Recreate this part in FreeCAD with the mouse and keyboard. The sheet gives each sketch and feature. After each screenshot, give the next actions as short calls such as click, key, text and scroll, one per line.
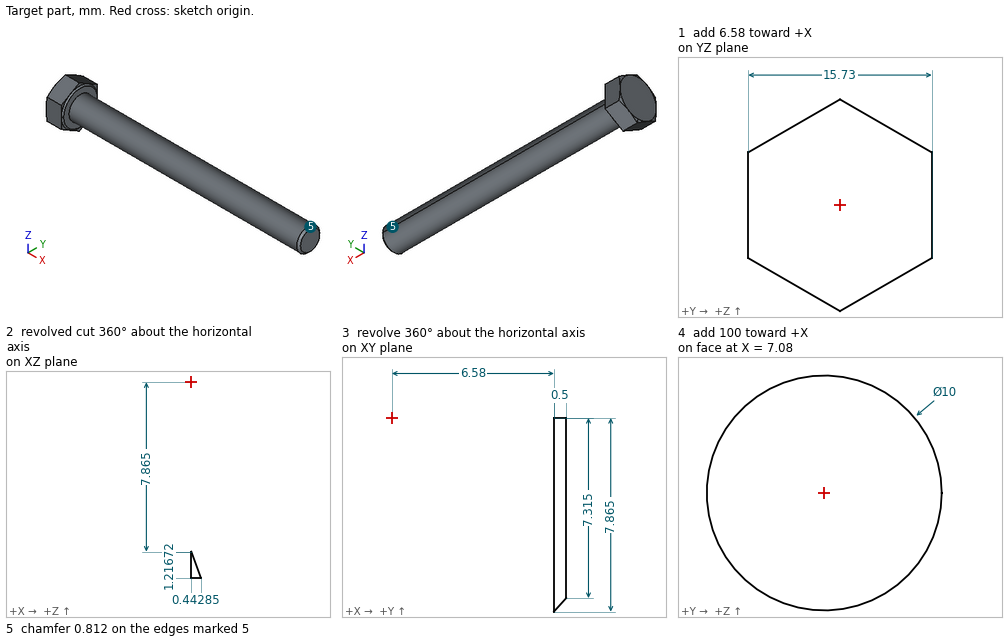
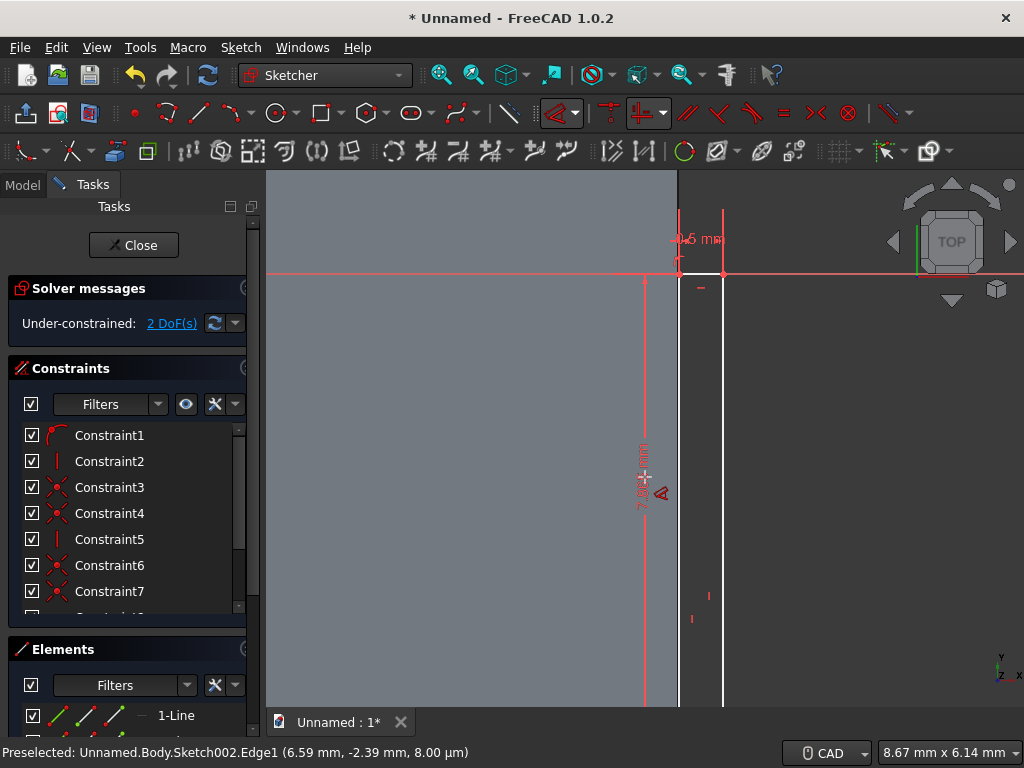
click(723, 467)
click(757, 477)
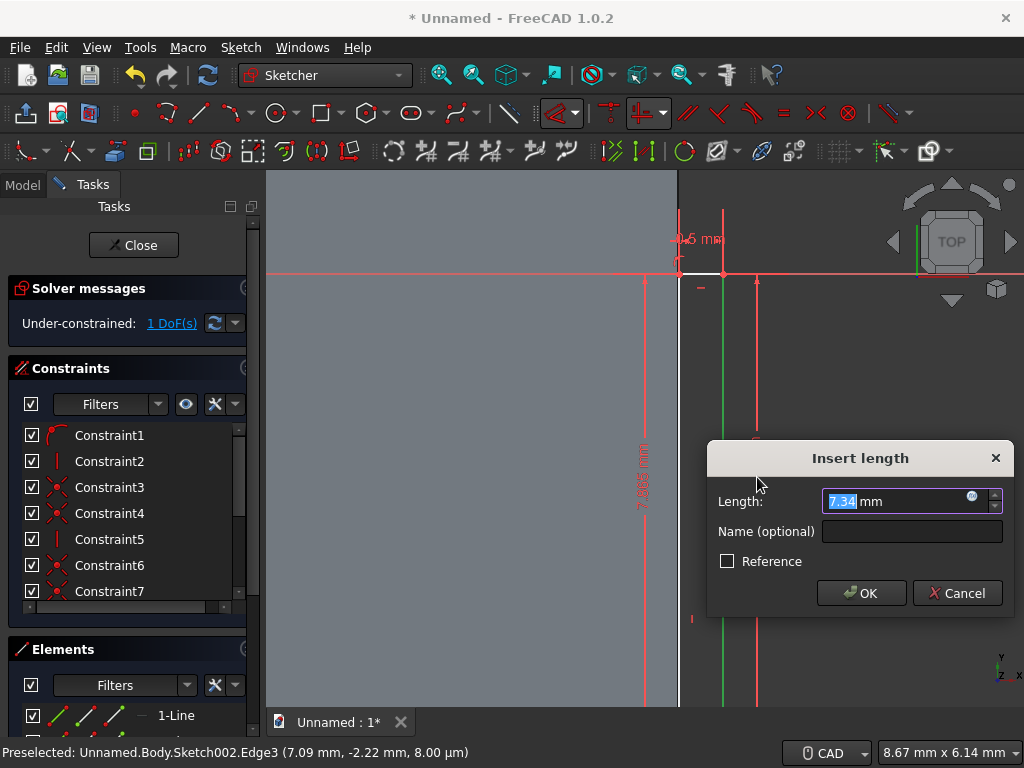
text(7.315)
key(Return)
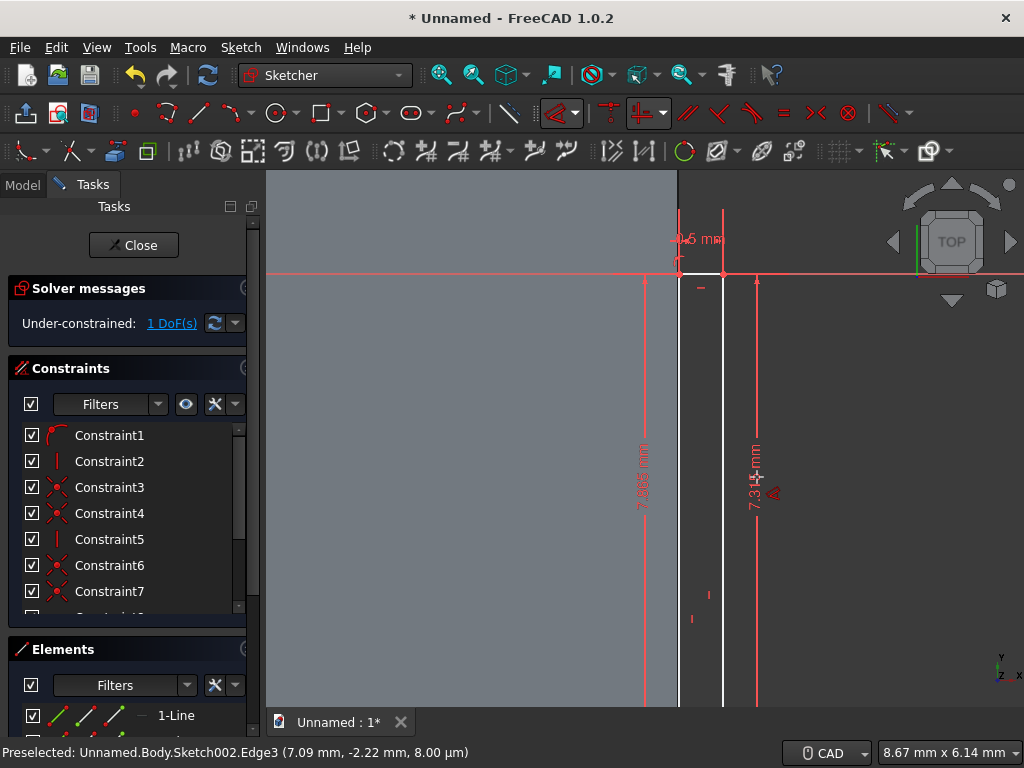
click(679, 274)
click(487, 240)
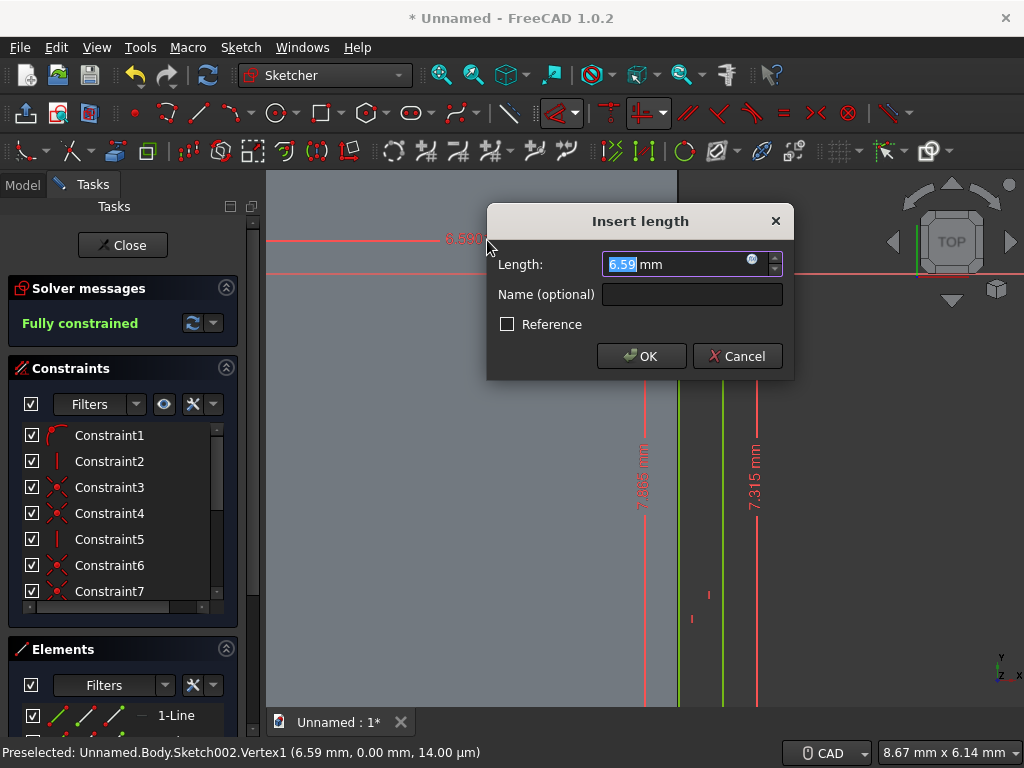
text(6.58)
key(Return)
key(Escape)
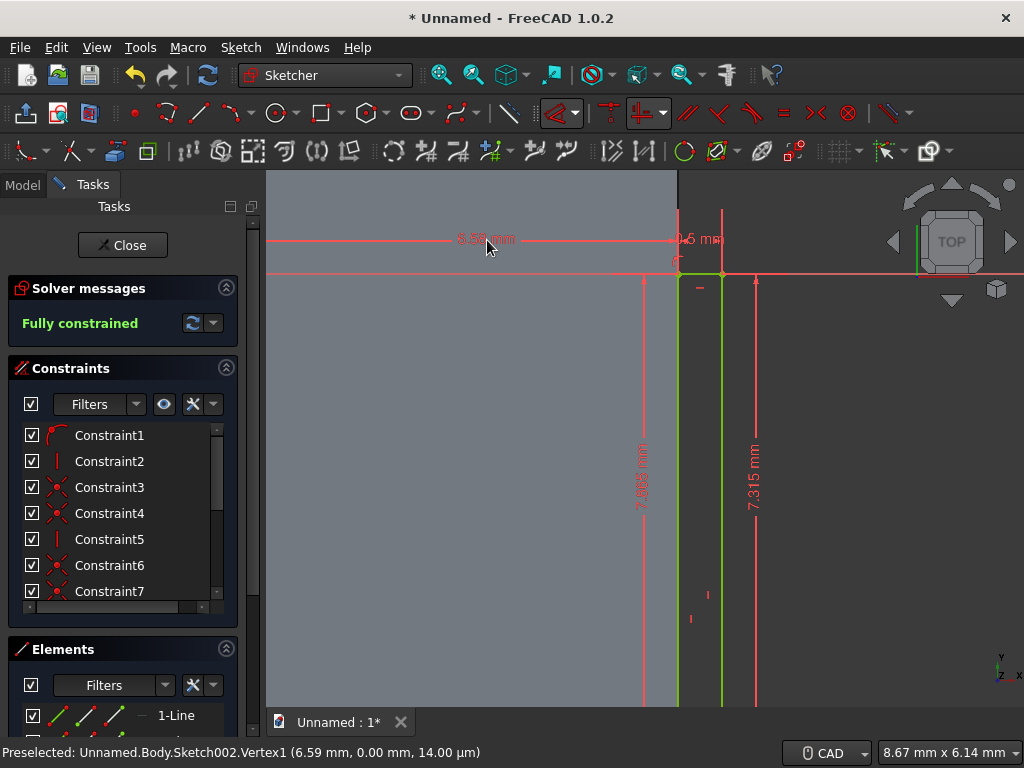
click(123, 245)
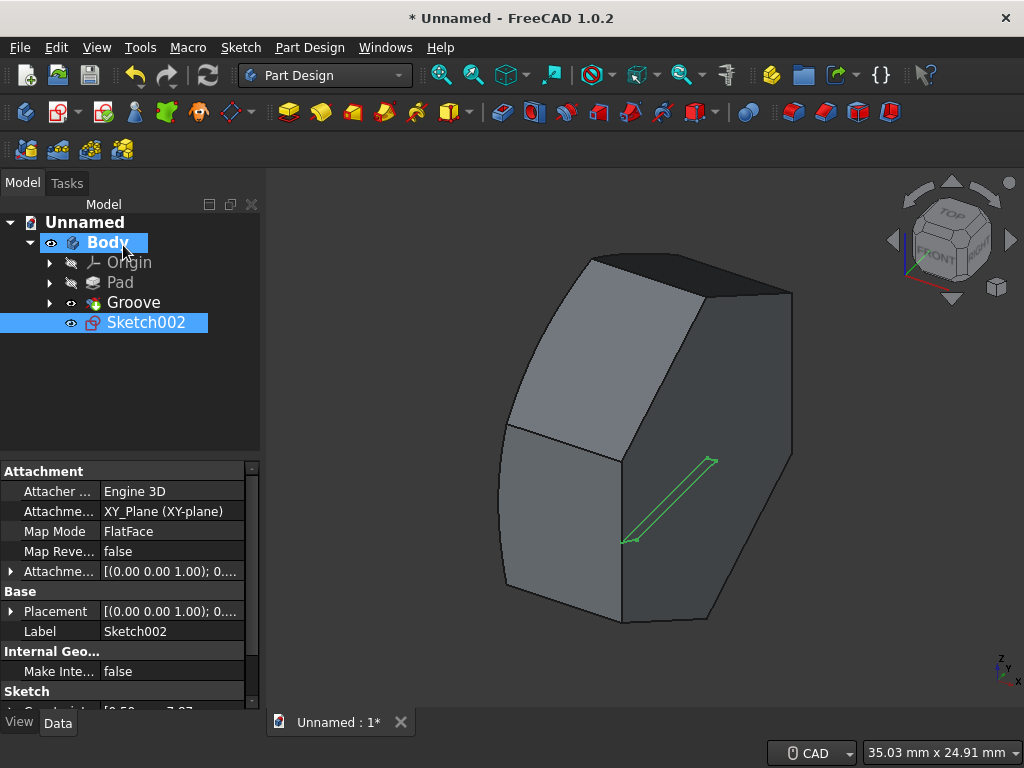
click(322, 112)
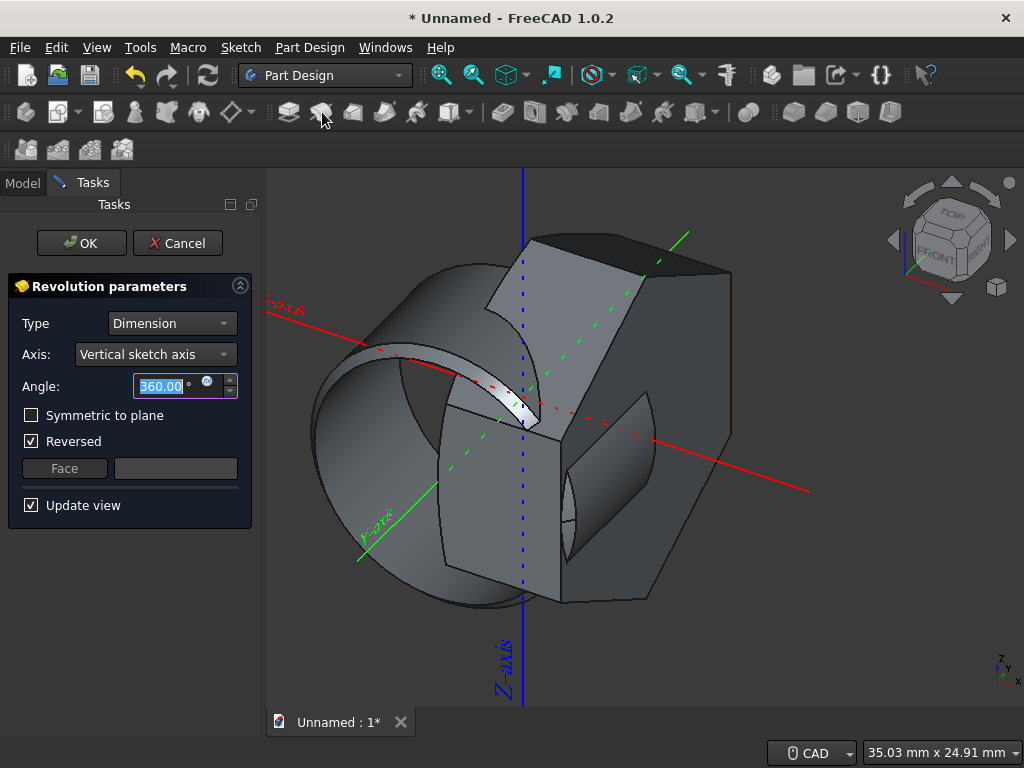
click(156, 354)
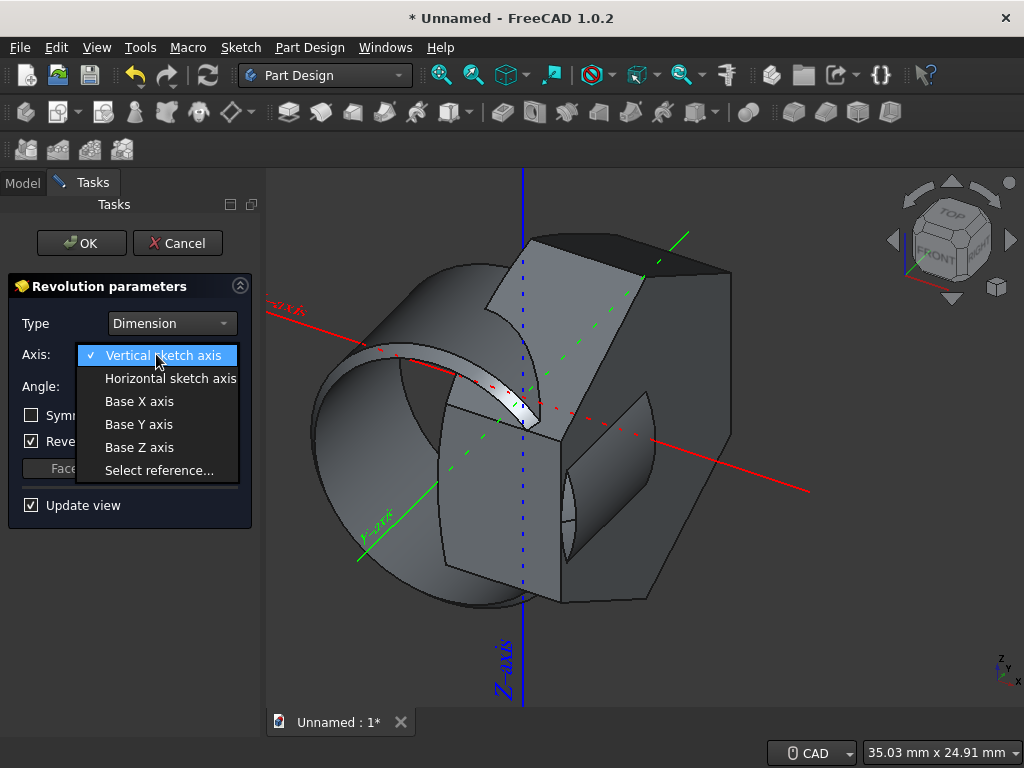
click(156, 378)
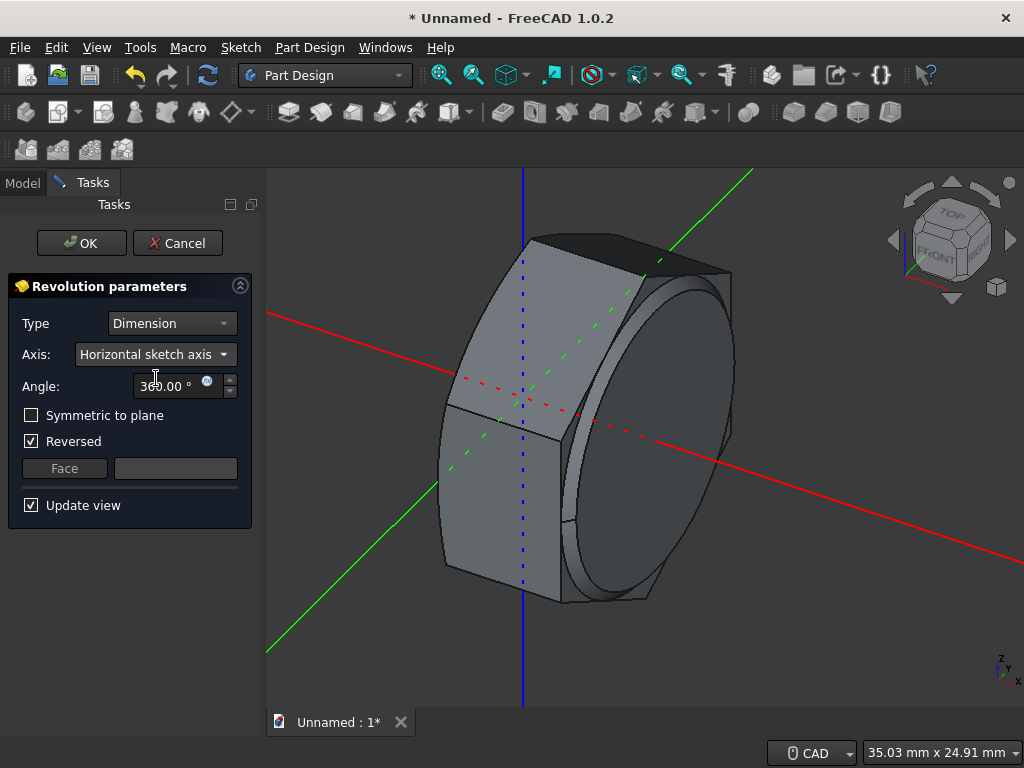
click(82, 243)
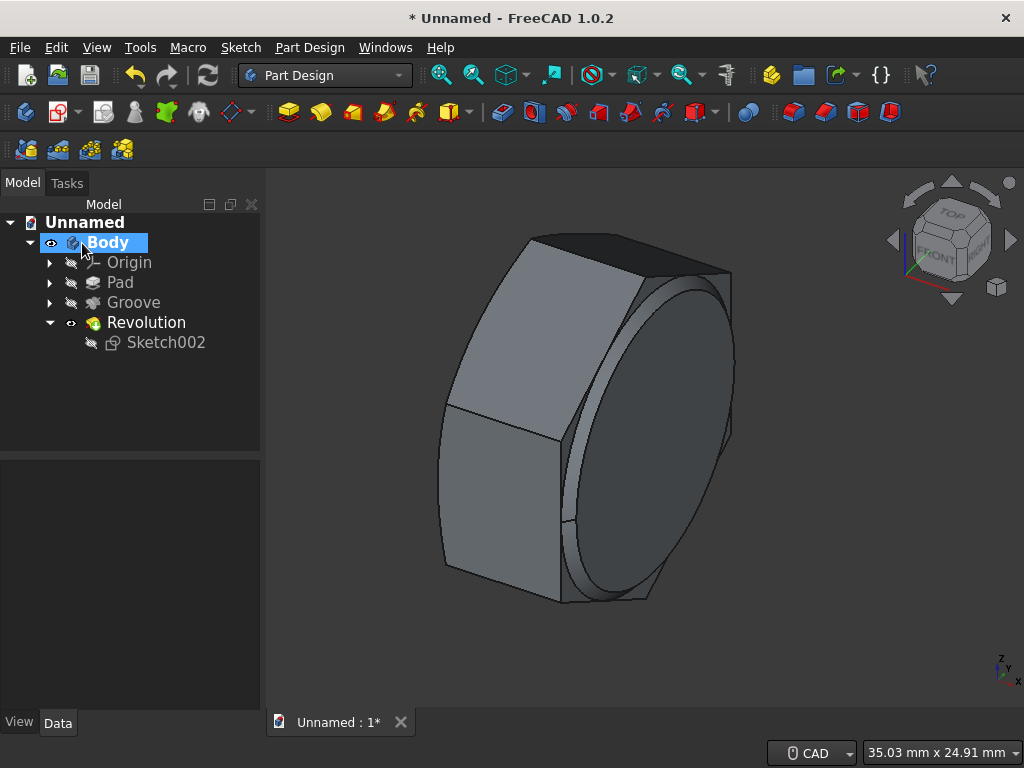
click(442, 76)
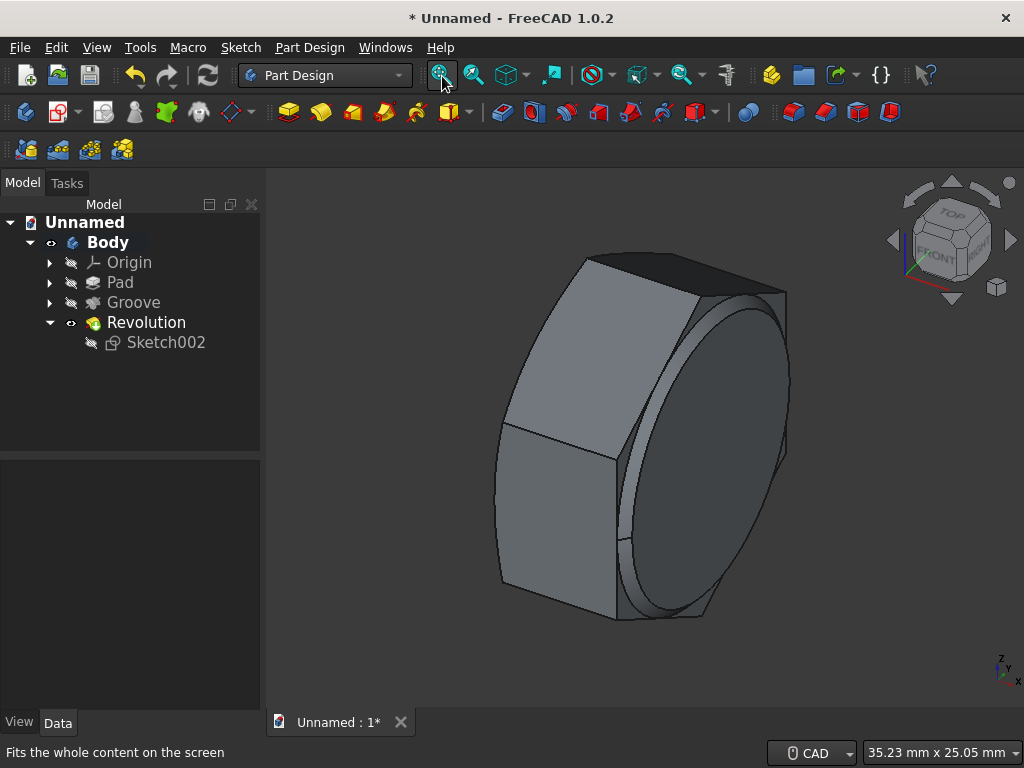
click(711, 458)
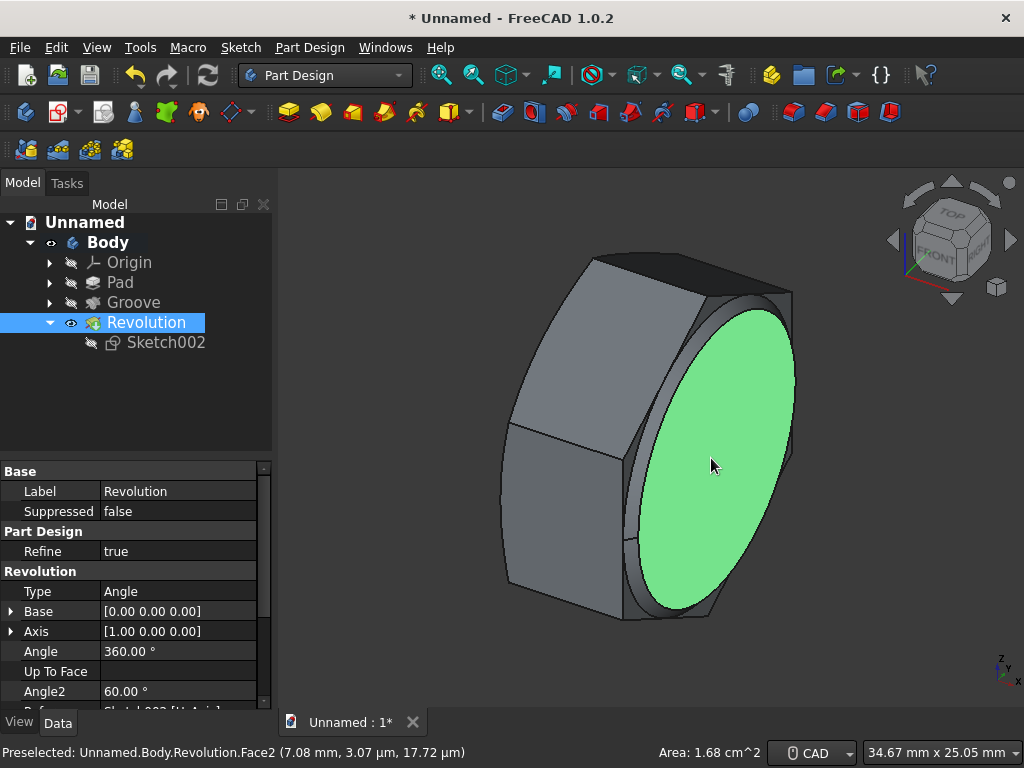
click(58, 112)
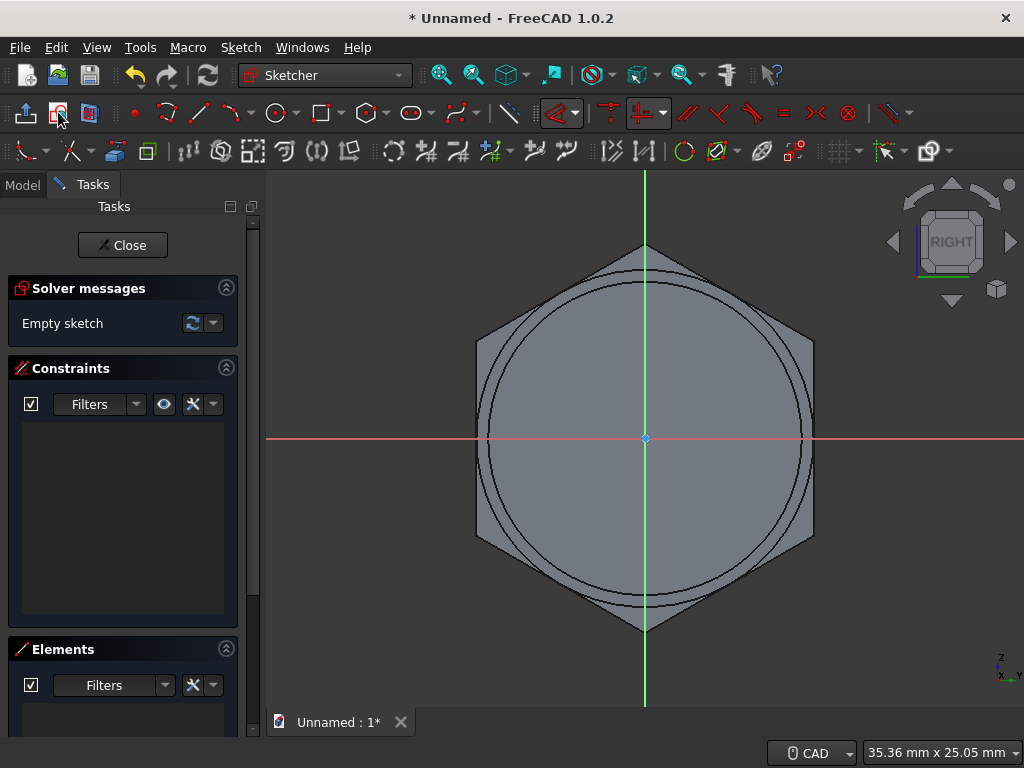
scroll(784, 438, up, 2)